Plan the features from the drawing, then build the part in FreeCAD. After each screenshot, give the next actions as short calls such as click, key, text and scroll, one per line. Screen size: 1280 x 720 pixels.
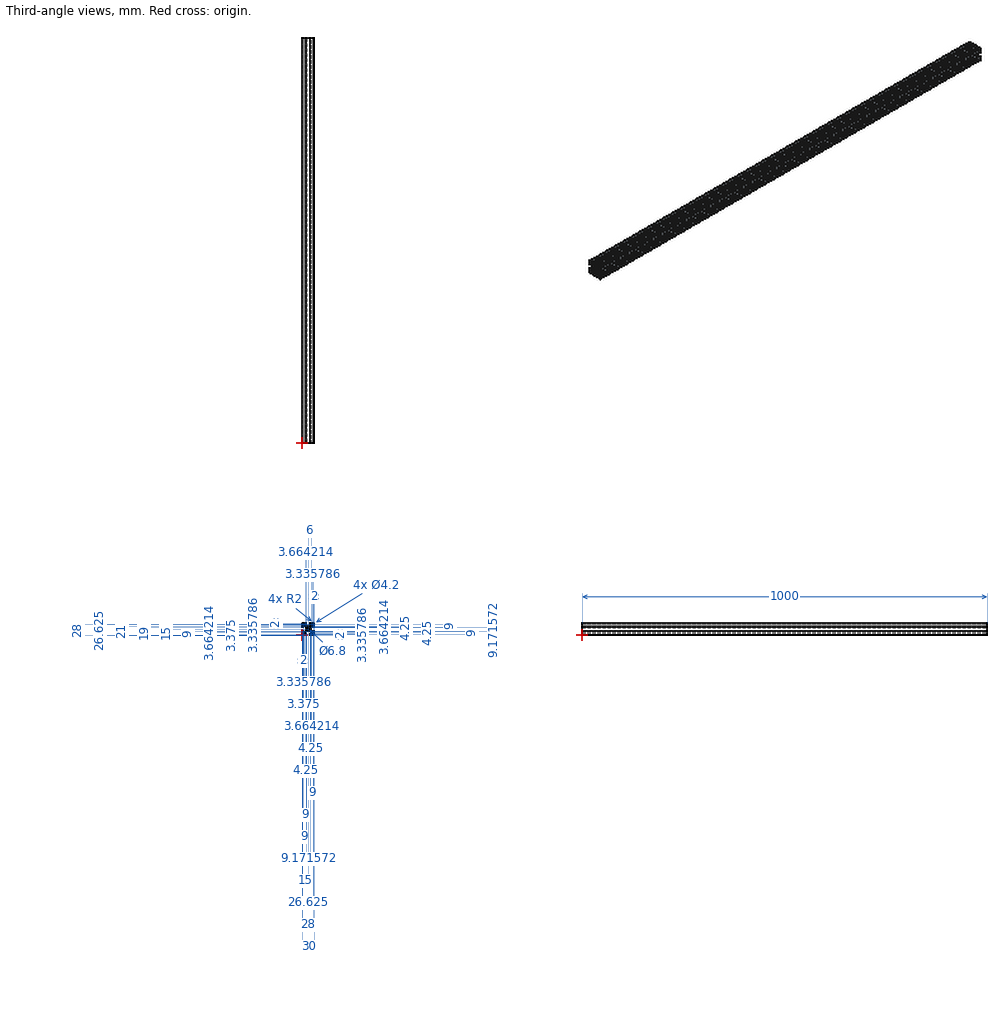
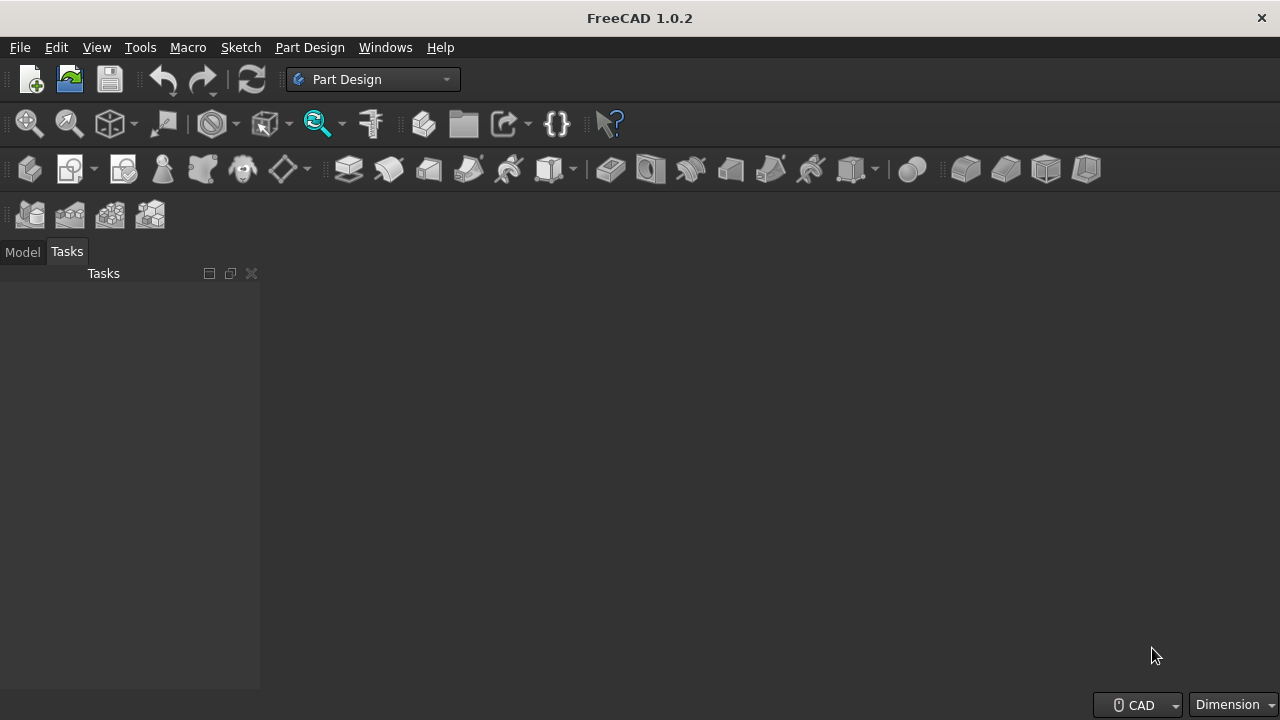
click(30, 80)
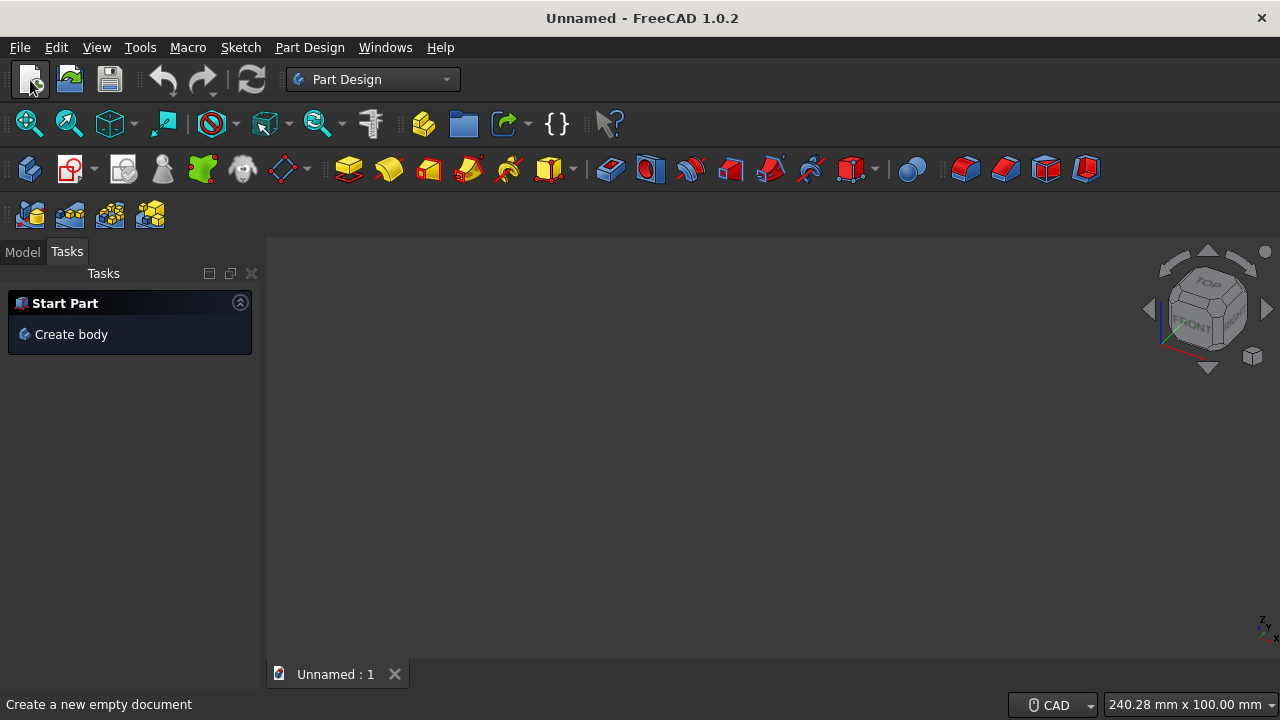
click(70, 170)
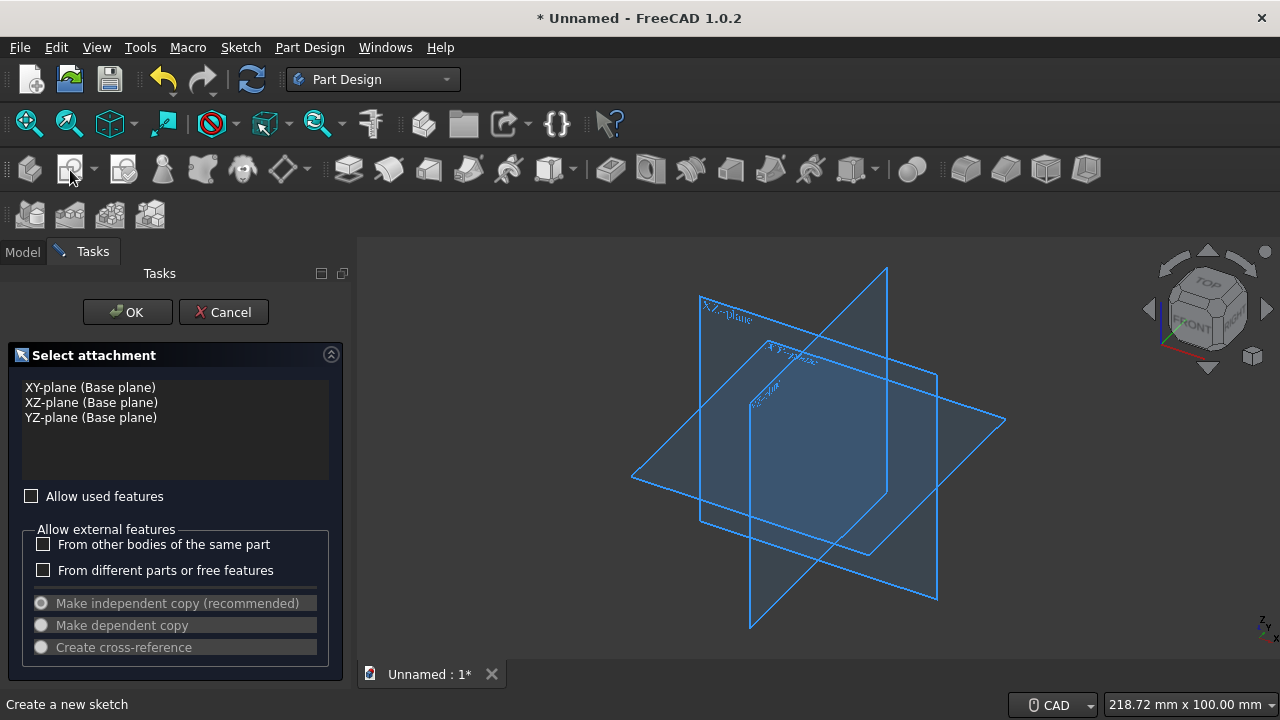
click(82, 402)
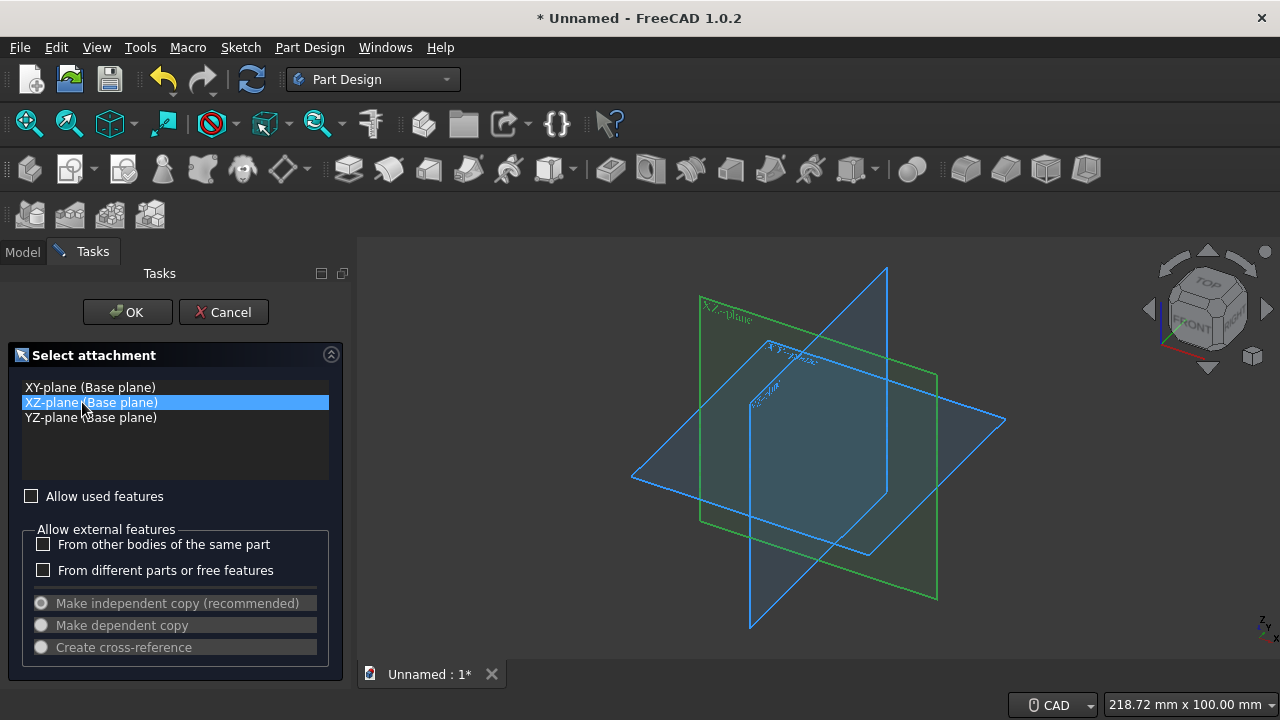
click(128, 312)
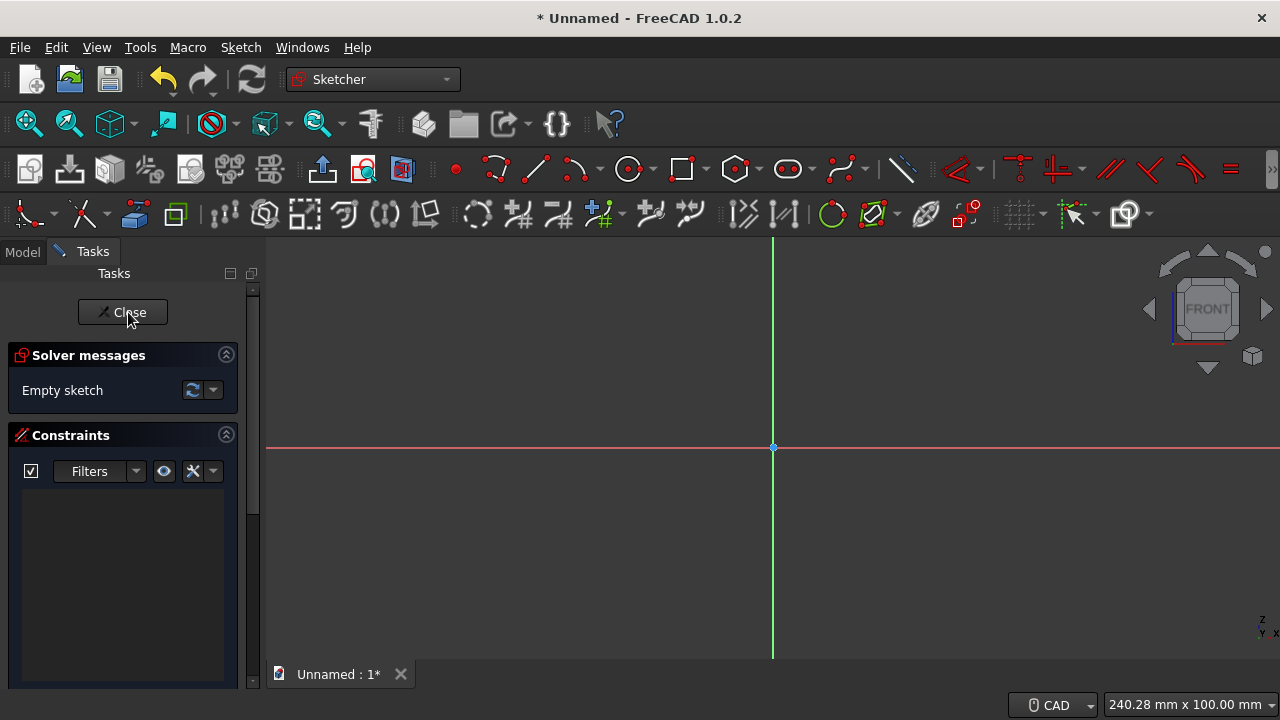
scroll(944, 333, up, 4)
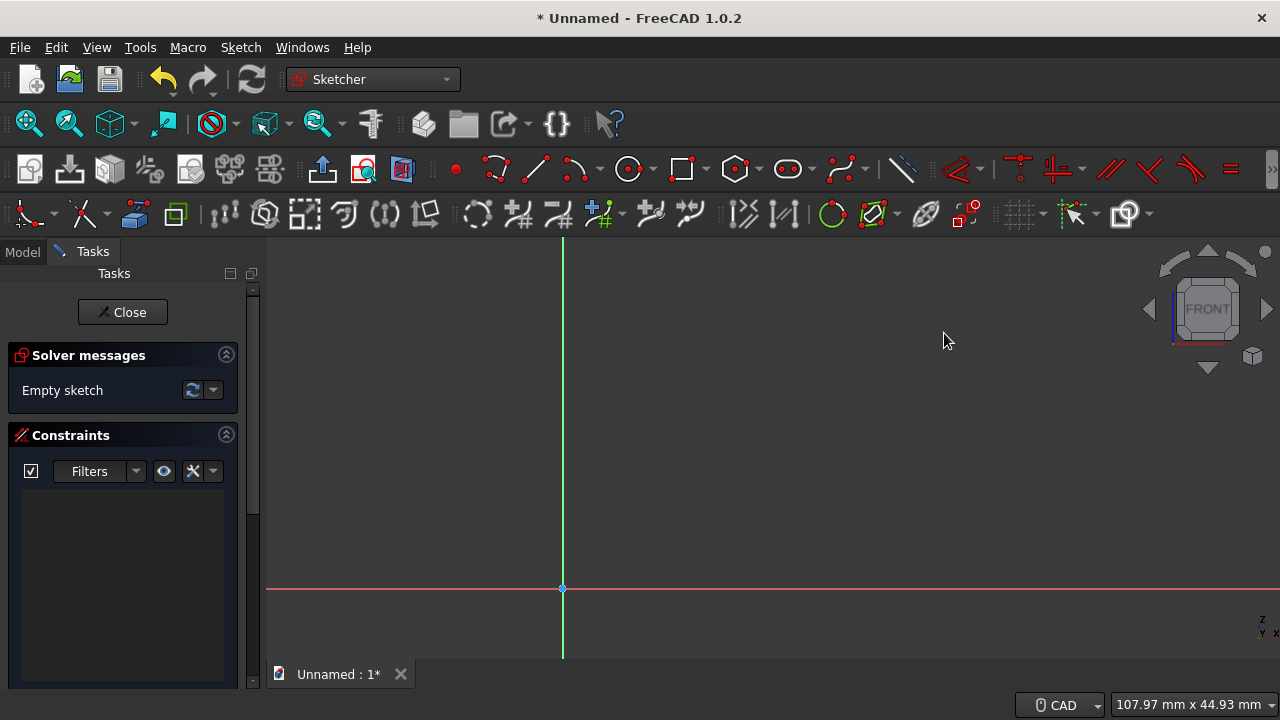
click(496, 170)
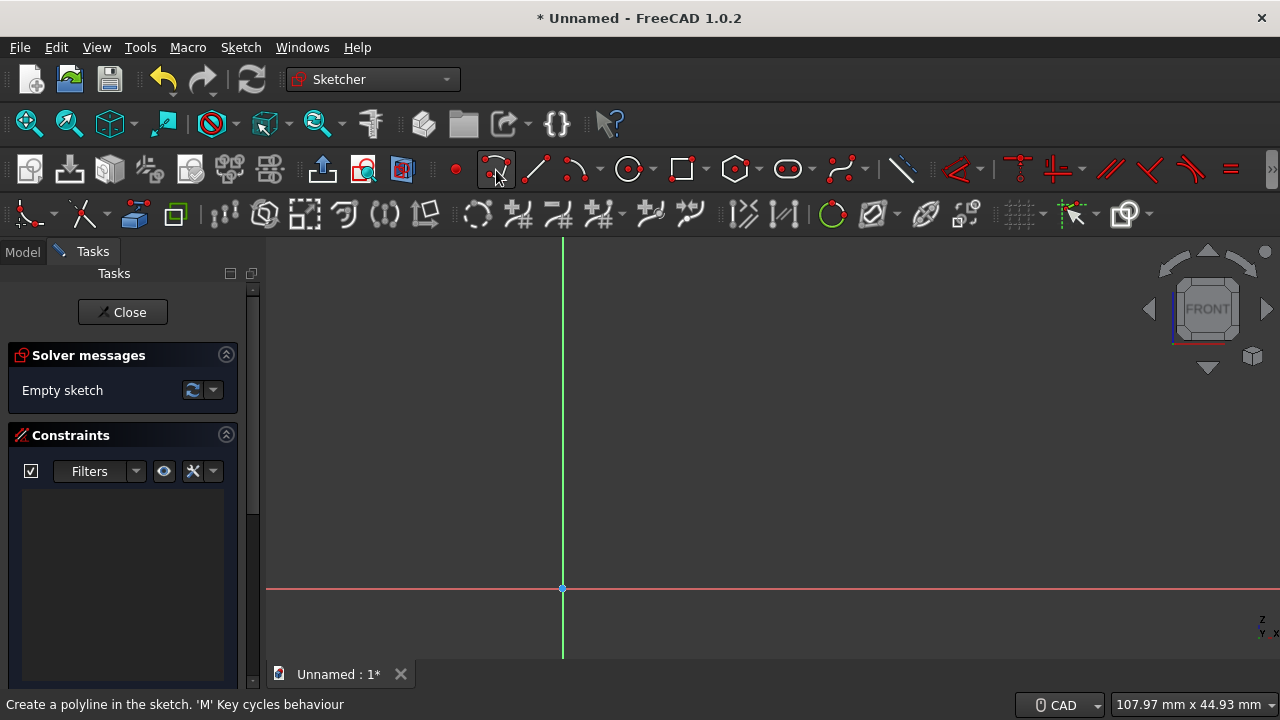
click(844, 326)
click(844, 410)
click(826, 410)
click(826, 370)
click(794, 370)
click(760, 405)
click(760, 491)
click(794, 525)
click(826, 525)
click(826, 485)
click(844, 485)
click(844, 570)
right_click(844, 570)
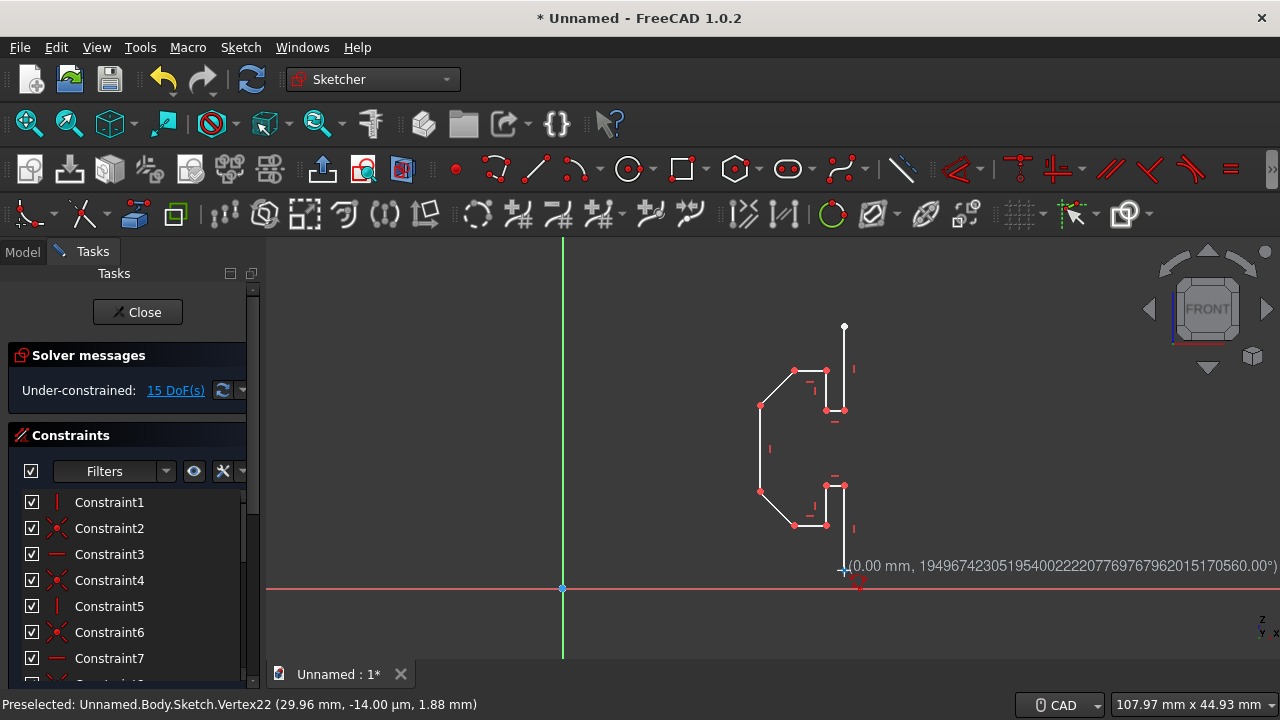
click(826, 589)
click(741, 580)
click(741, 570)
click(781, 570)
click(781, 539)
click(747, 504)
click(660, 504)
click(626, 539)
click(626, 570)
click(666, 570)
click(666, 589)
click(581, 580)
right_click(581, 580)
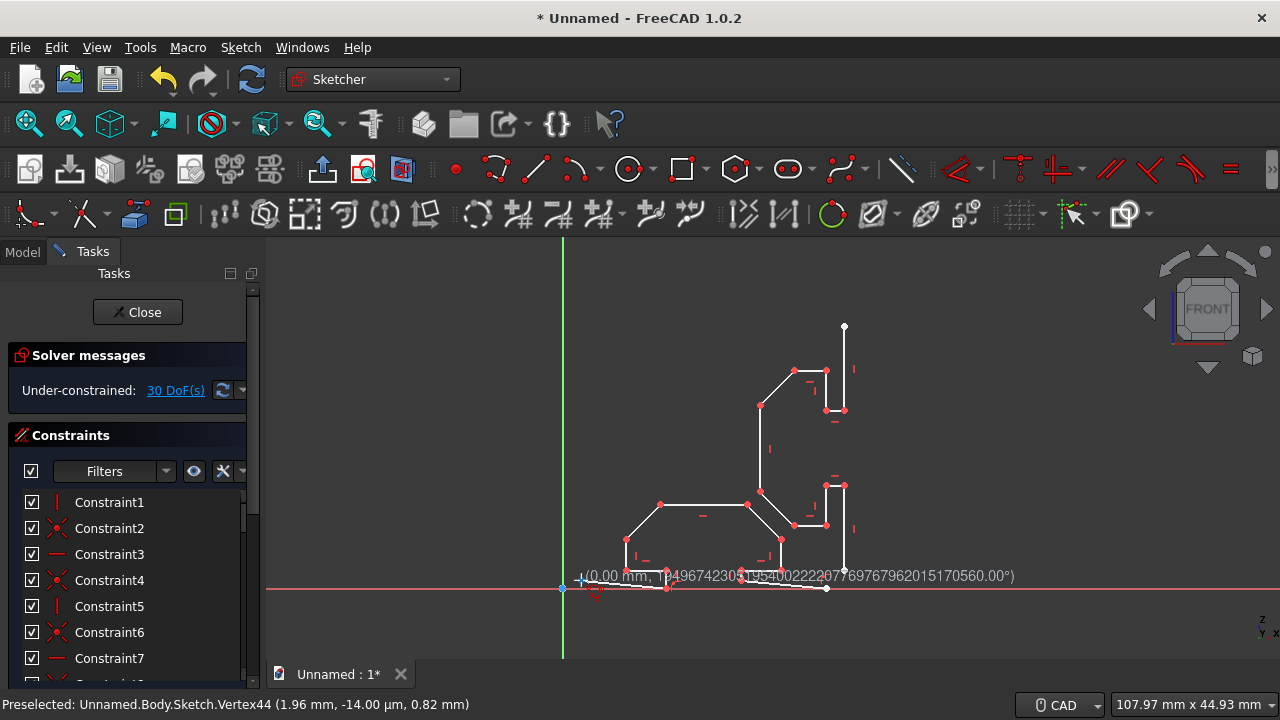
click(563, 570)
click(572, 485)
click(581, 485)
click(581, 525)
click(613, 525)
click(647, 491)
click(647, 405)
click(613, 370)
click(581, 370)
click(581, 410)
click(563, 410)
click(572, 326)
right_click(572, 326)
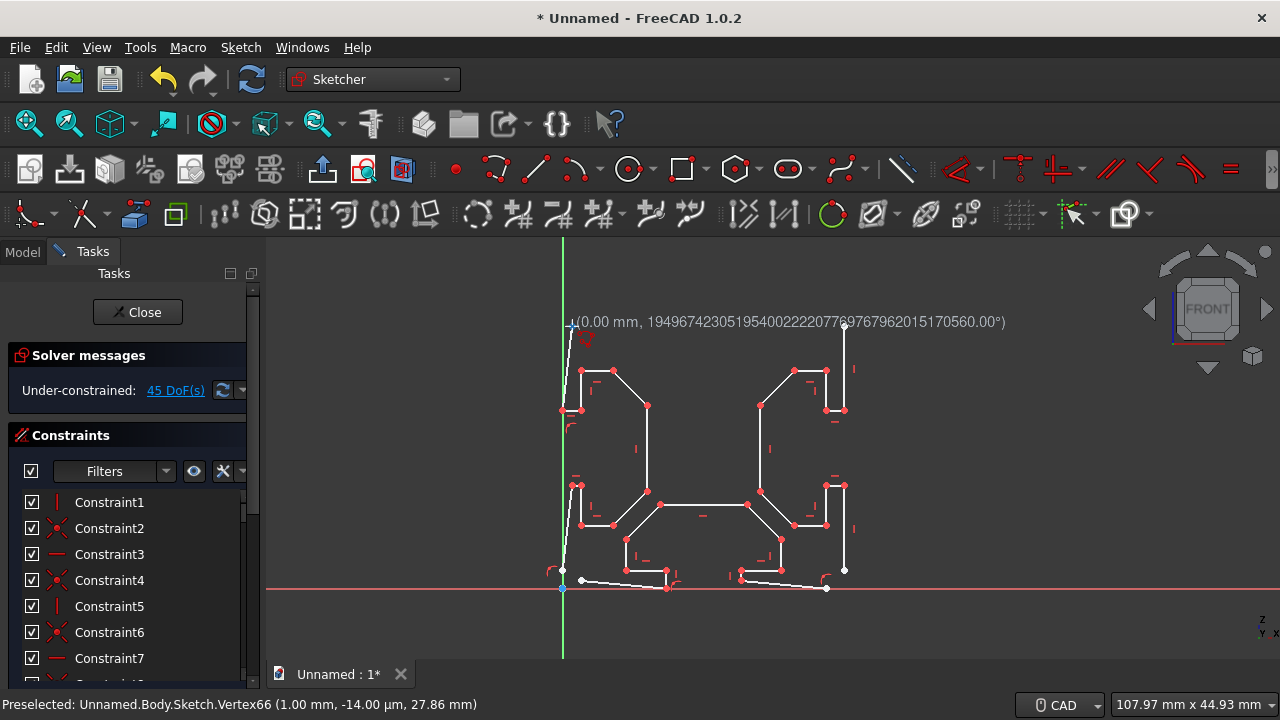
click(581, 307)
click(666, 307)
click(666, 326)
click(626, 326)
click(626, 357)
click(660, 391)
click(747, 391)
click(781, 357)
click(781, 326)
click(741, 326)
click(741, 307)
click(826, 307)
right_click(826, 307)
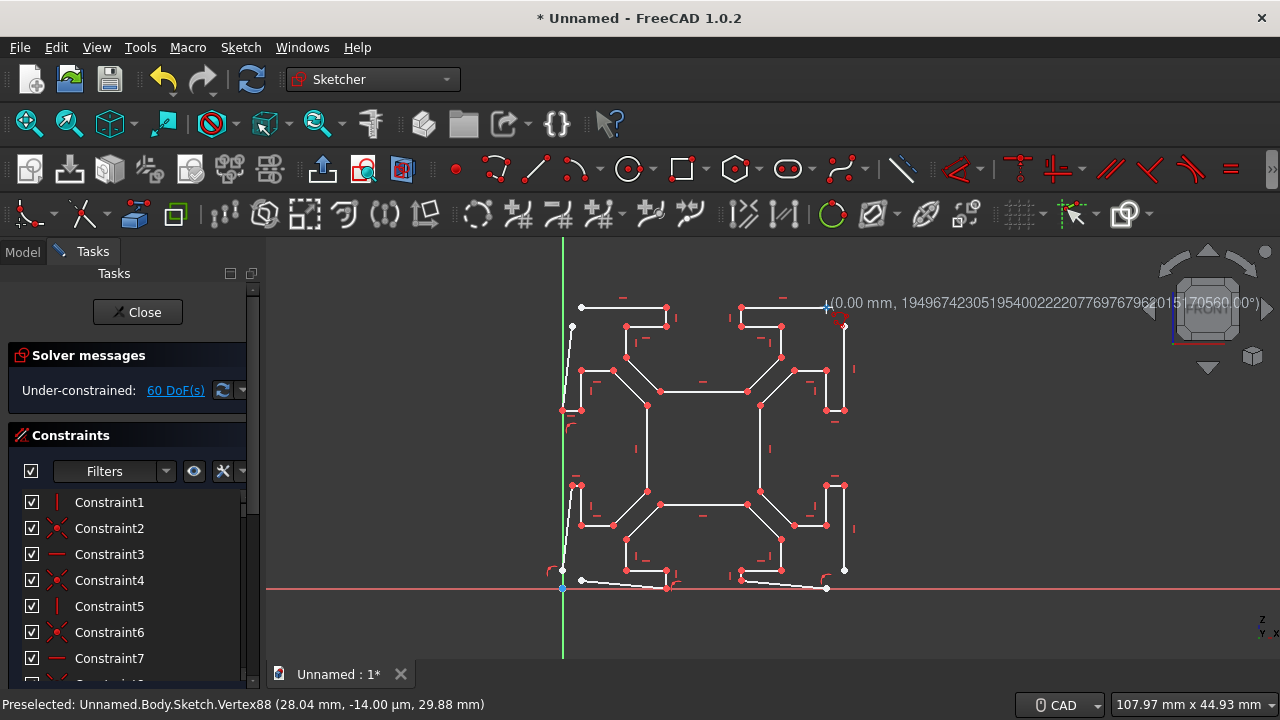
click(602, 170)